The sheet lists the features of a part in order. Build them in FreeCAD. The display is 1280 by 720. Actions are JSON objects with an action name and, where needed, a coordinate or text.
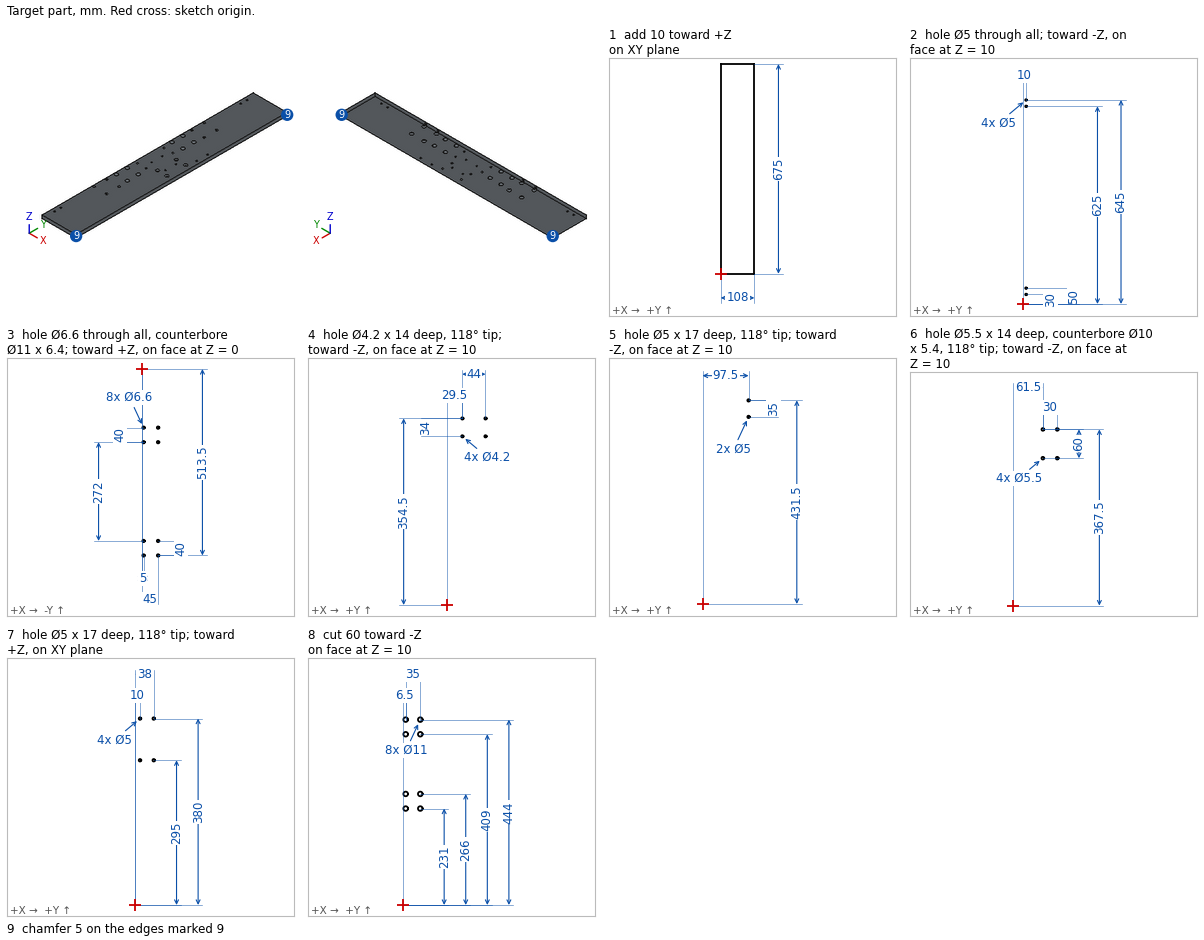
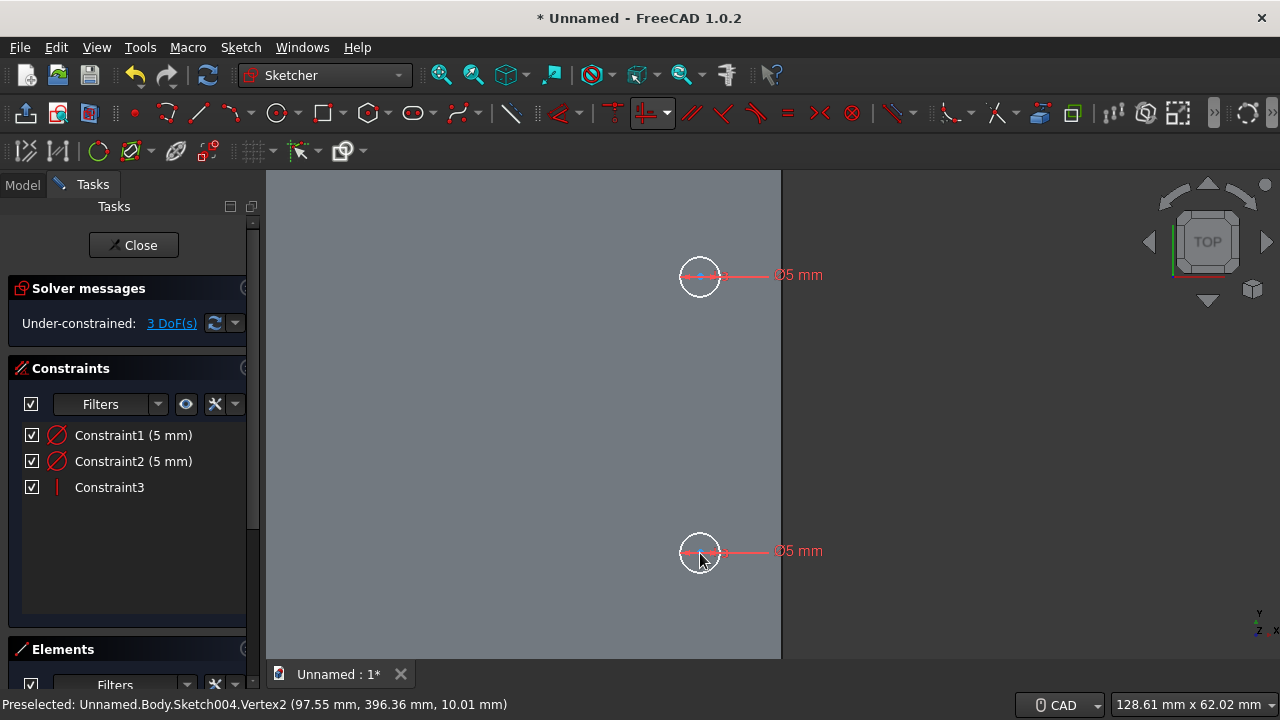
{"action": "left_click", "coordinate": [558, 114]}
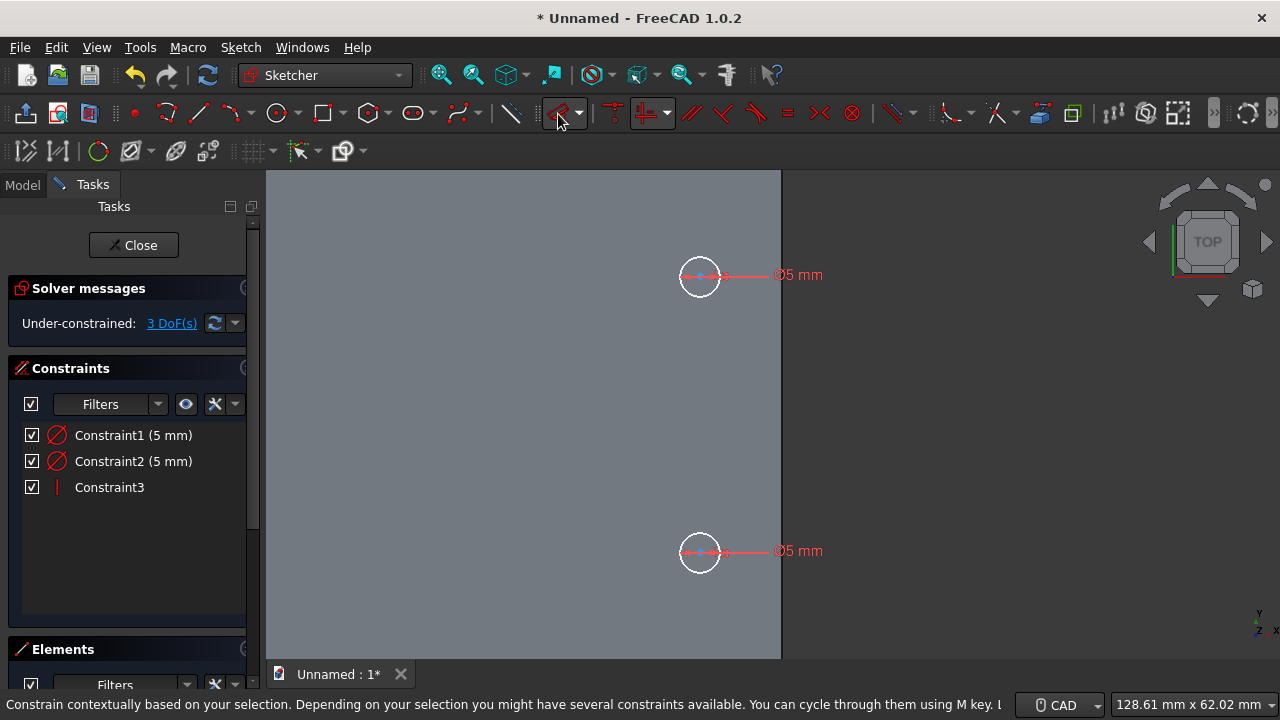
{"action": "left_click", "coordinate": [700, 277]}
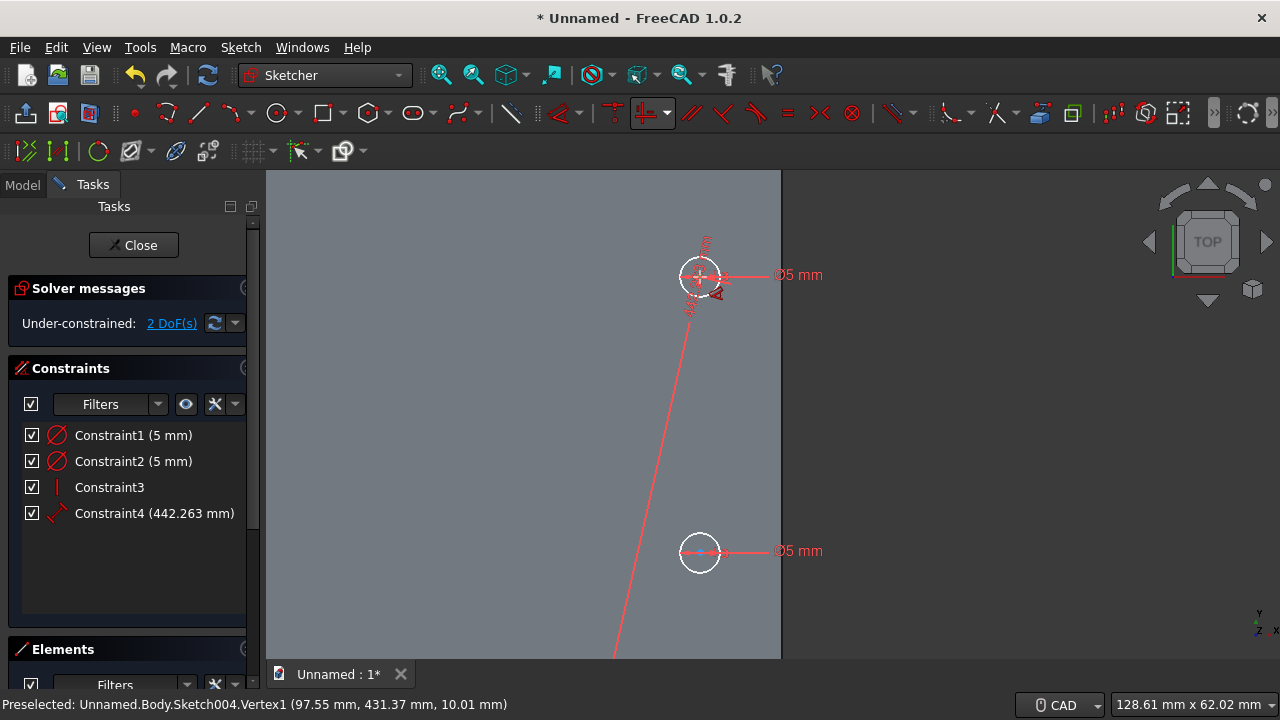
{"action": "left_click", "coordinate": [700, 553]}
{"action": "left_click", "coordinate": [734, 415]}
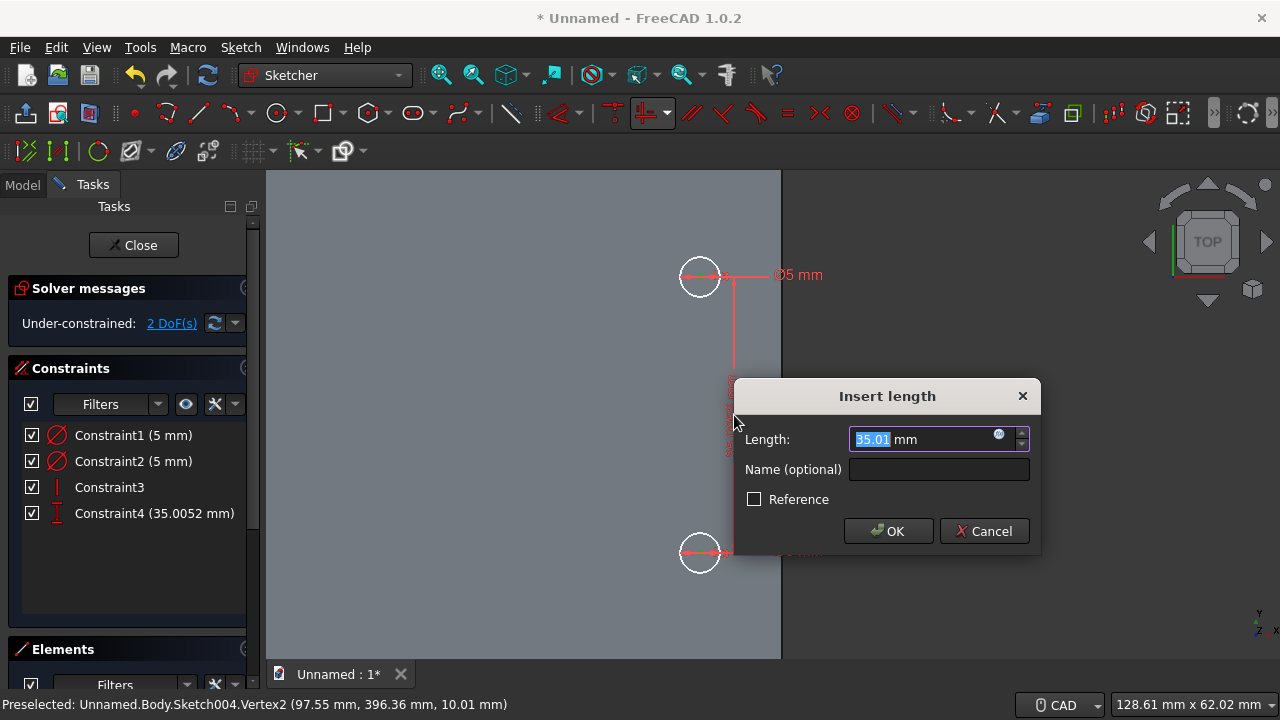
{"action": "type", "text": "35"}
{"action": "key", "text": "Return"}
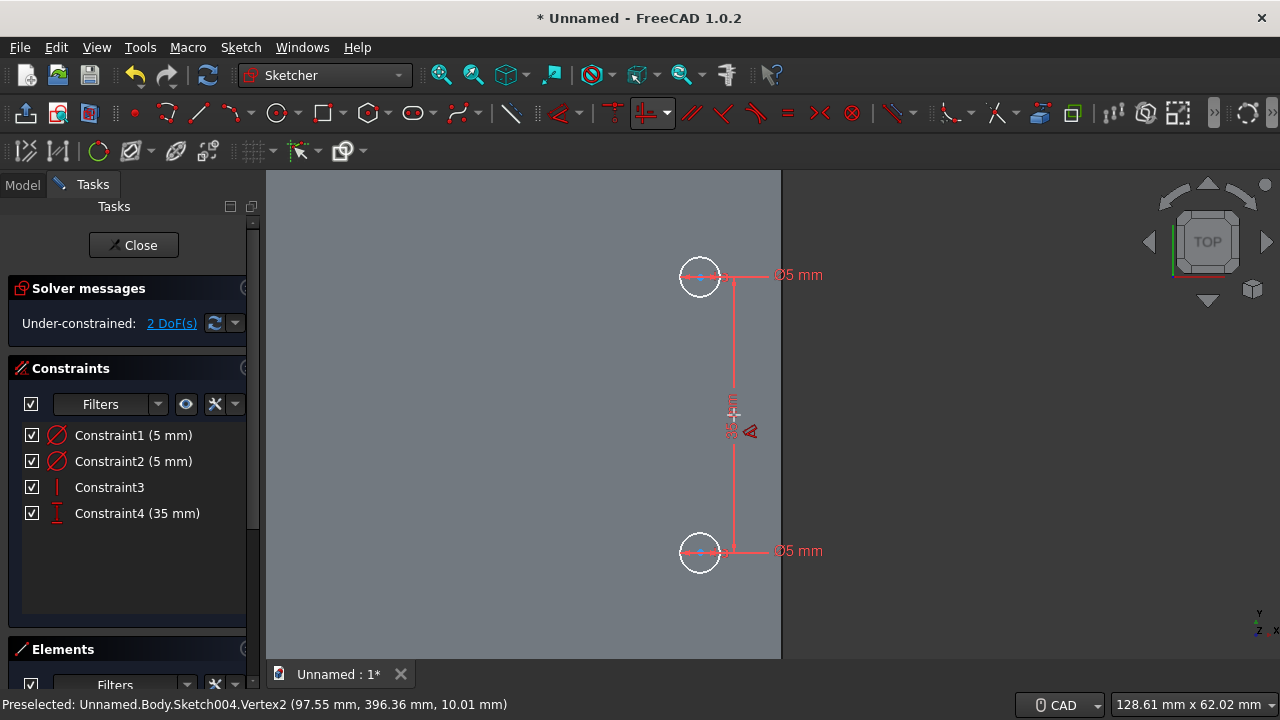
{"action": "left_click", "coordinate": [700, 277]}
{"action": "left_click", "coordinate": [497, 243]}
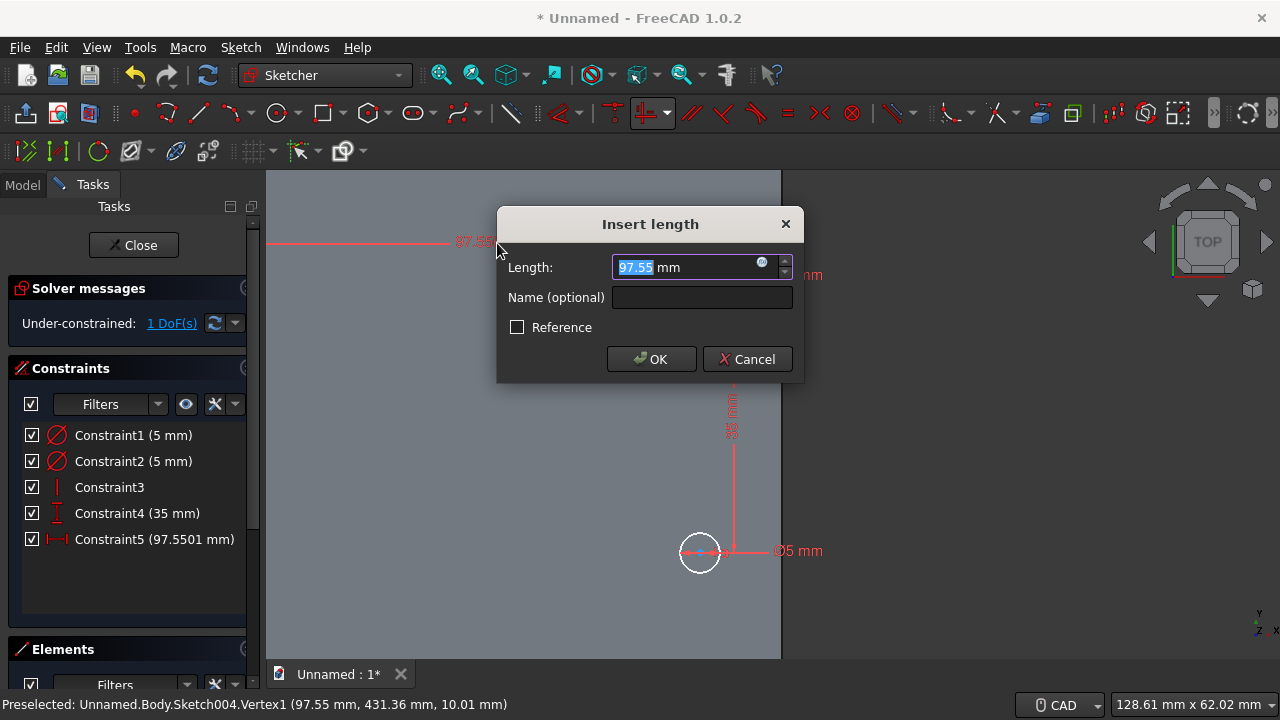
{"action": "type", "text": "97.5"}
{"action": "key", "text": "Return"}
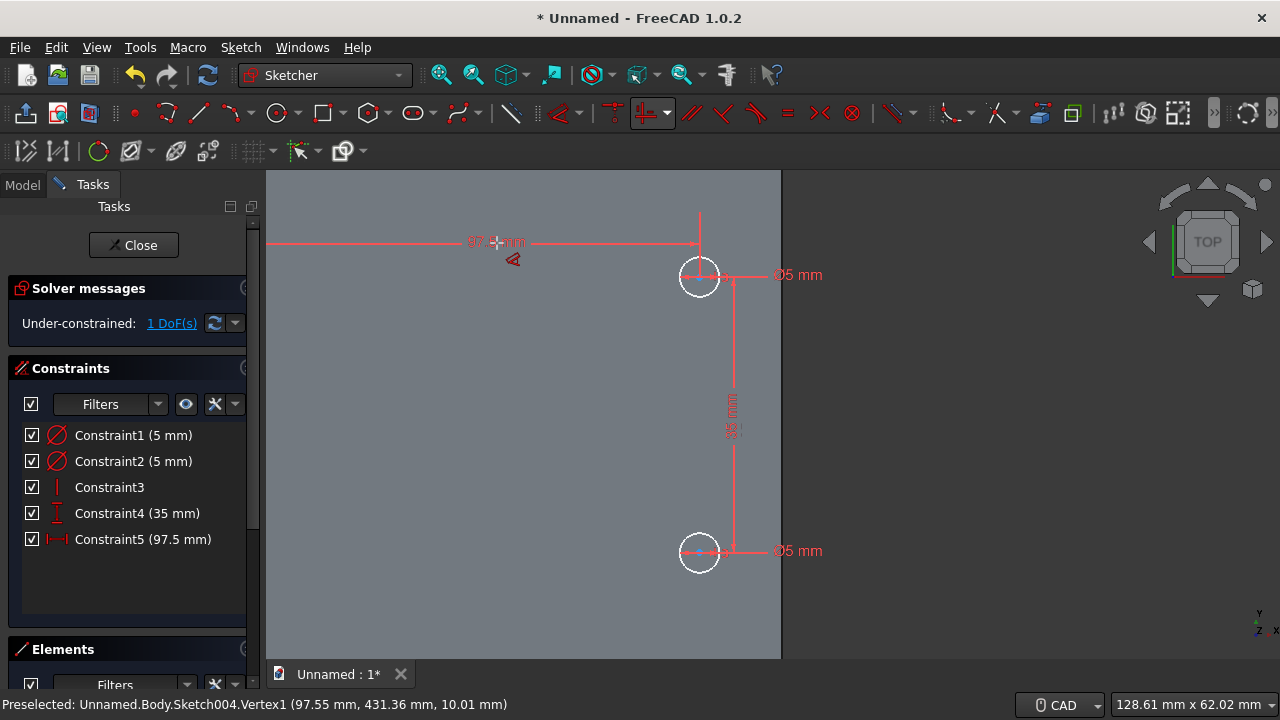
{"action": "left_click", "coordinate": [700, 277]}
{"action": "left_click", "coordinate": [734, 454]}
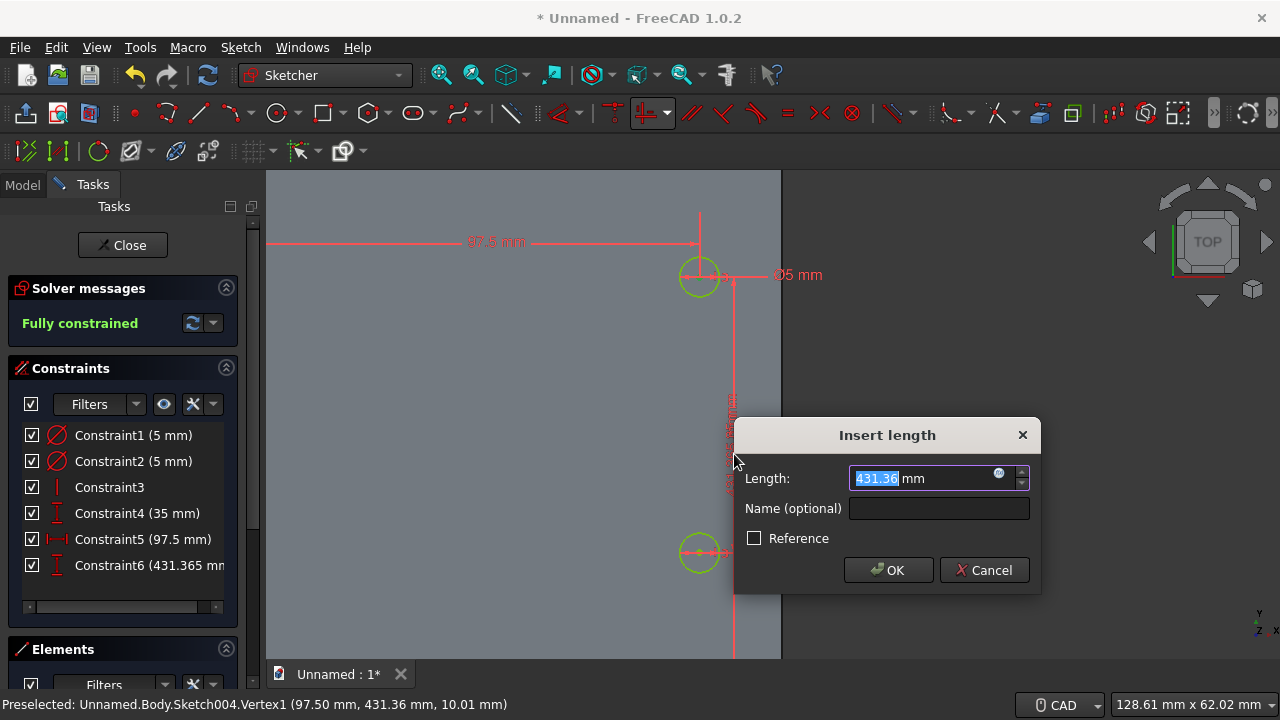
{"action": "type", "text": "431.5"}
{"action": "key", "text": "Return"}
{"action": "key", "text": "Escape"}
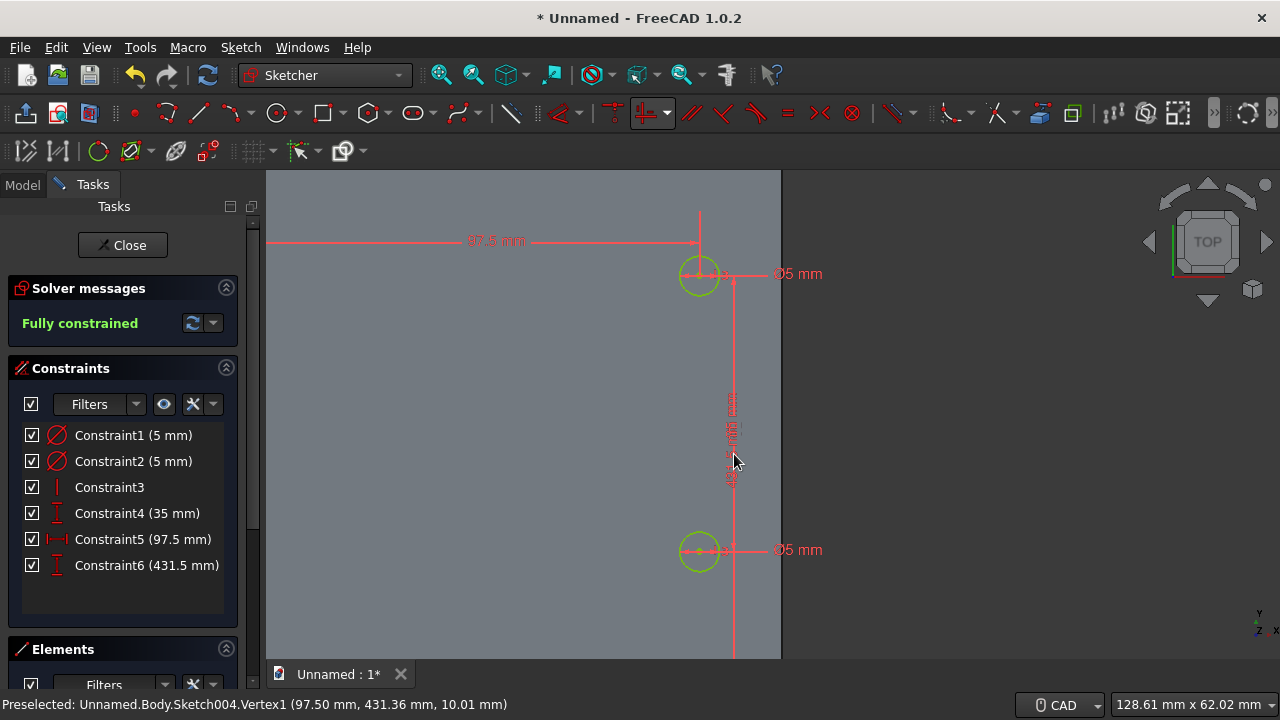
{"action": "left_click", "coordinate": [123, 245]}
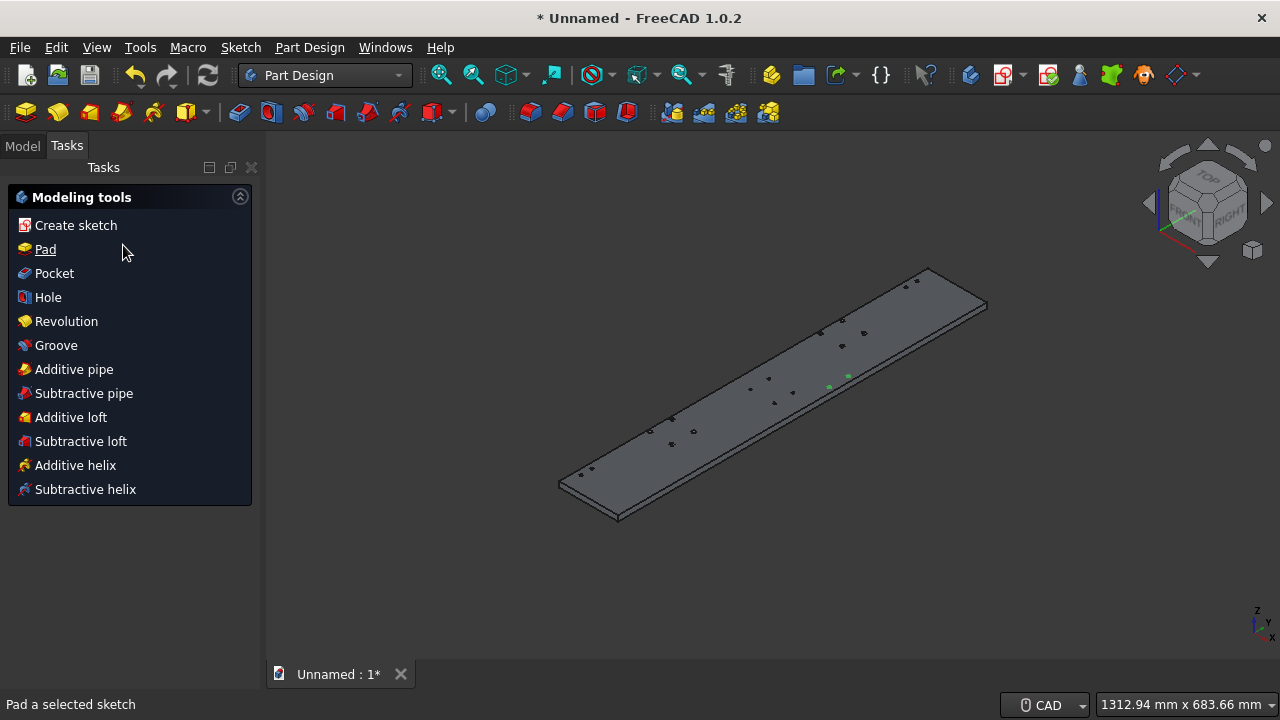
{"action": "left_click", "coordinate": [272, 112]}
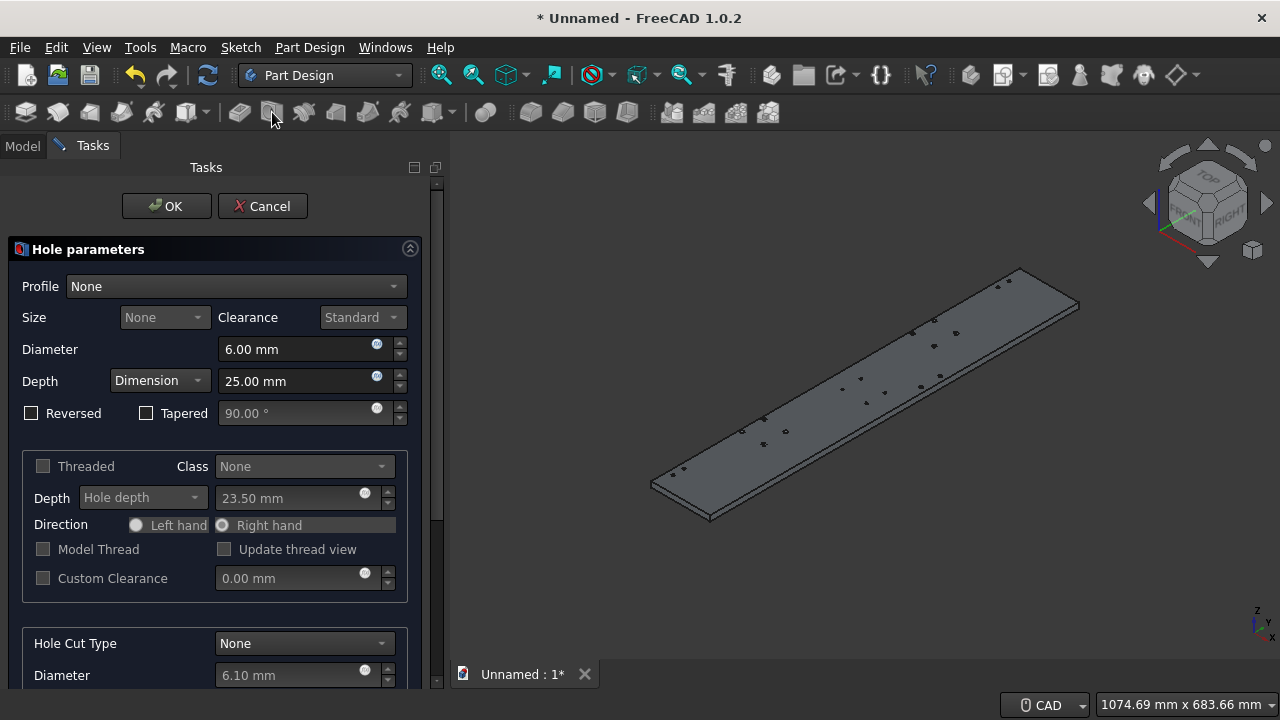
{"action": "triple_click", "coordinate": [305, 349]}